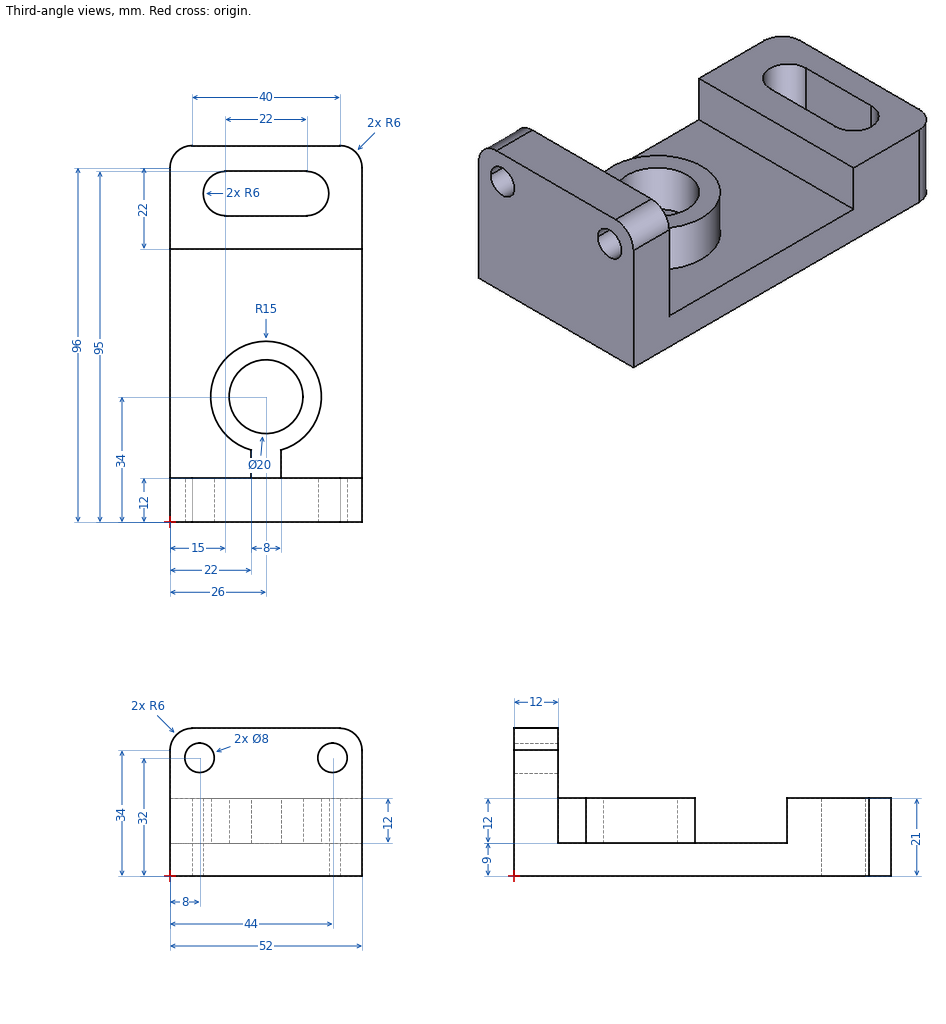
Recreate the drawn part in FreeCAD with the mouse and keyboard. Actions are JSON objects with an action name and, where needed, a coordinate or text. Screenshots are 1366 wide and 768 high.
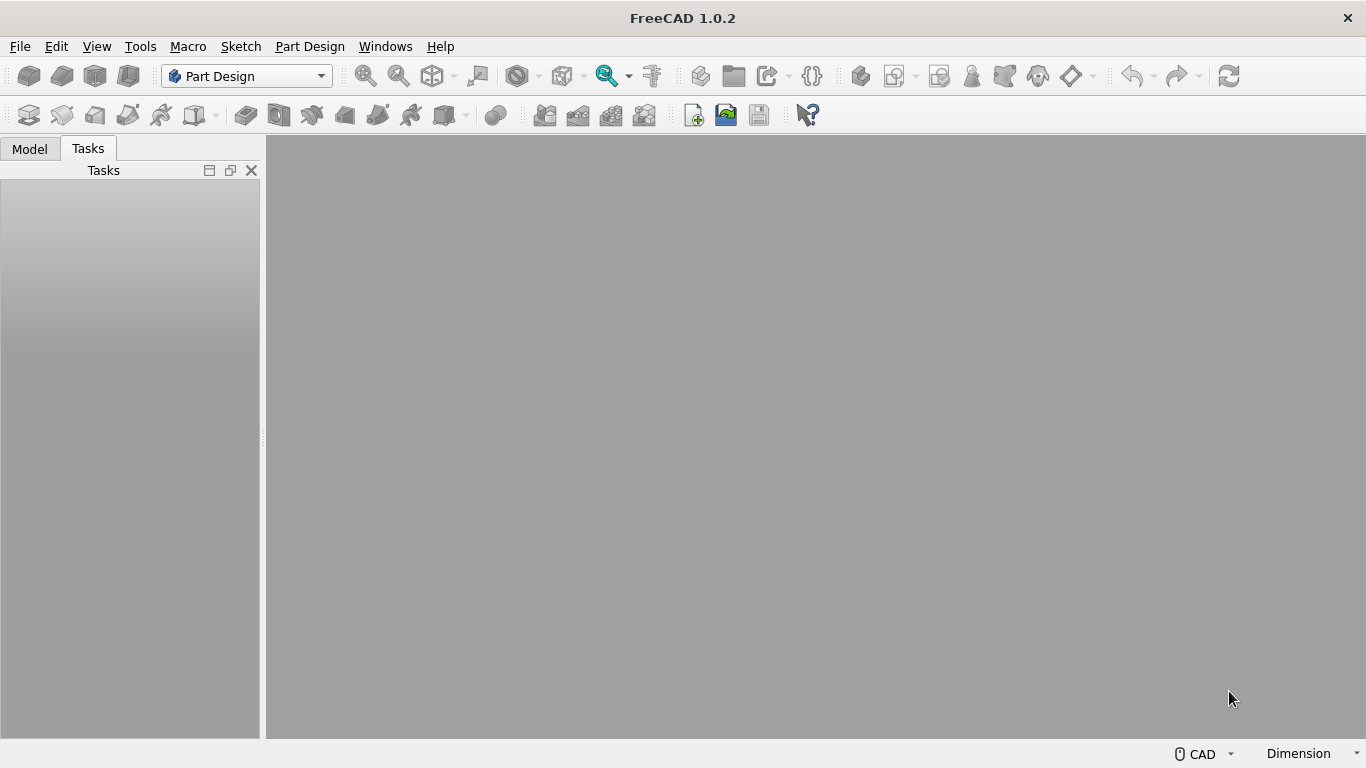
{"action": "left_click", "coordinate": [693, 116]}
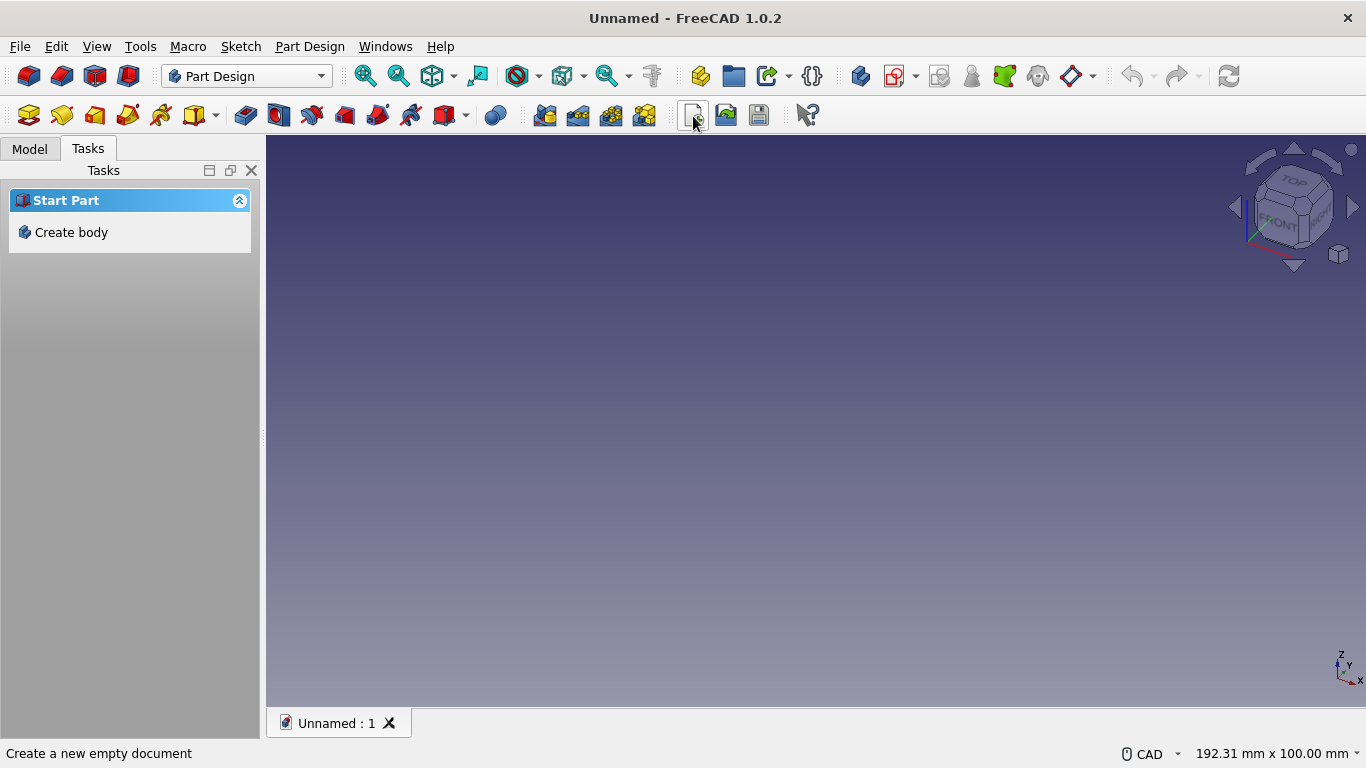
{"action": "left_click", "coordinate": [894, 76]}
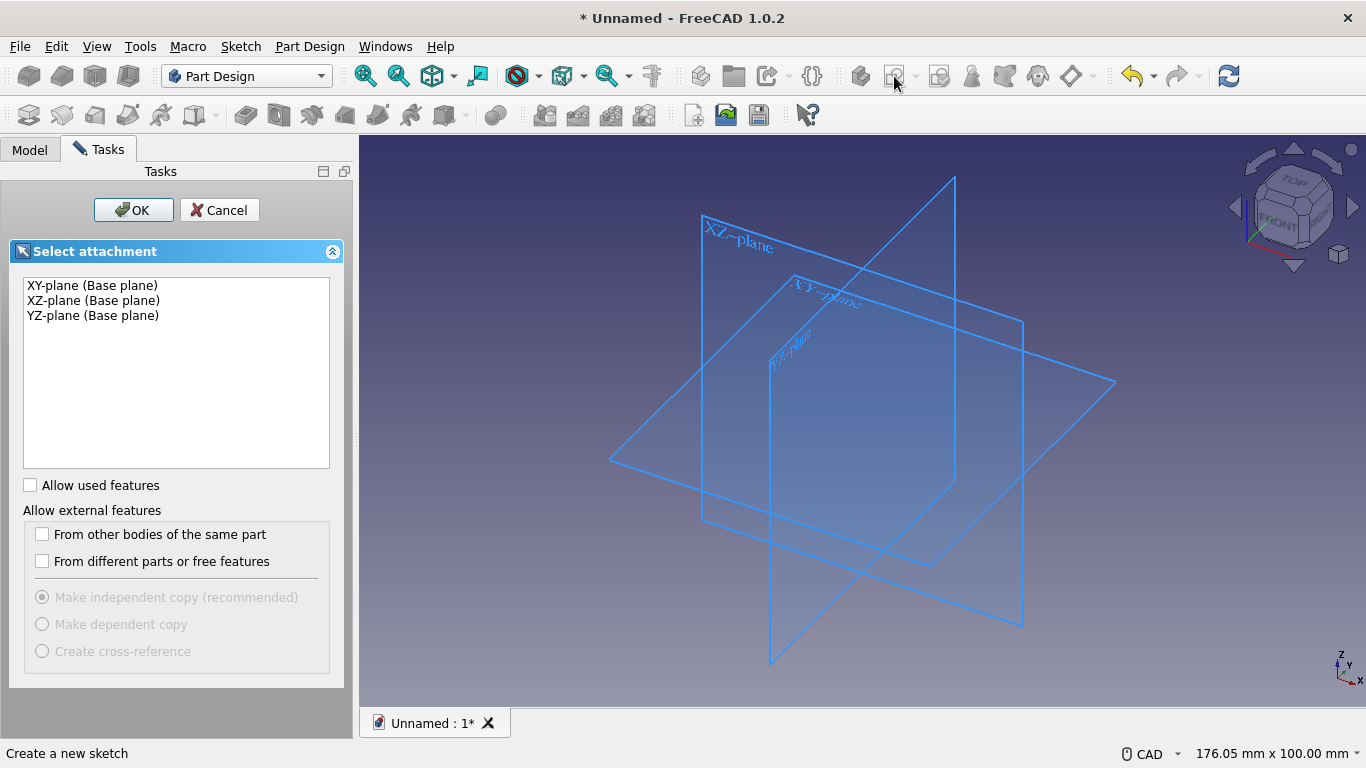
{"action": "left_click", "coordinate": [84, 286]}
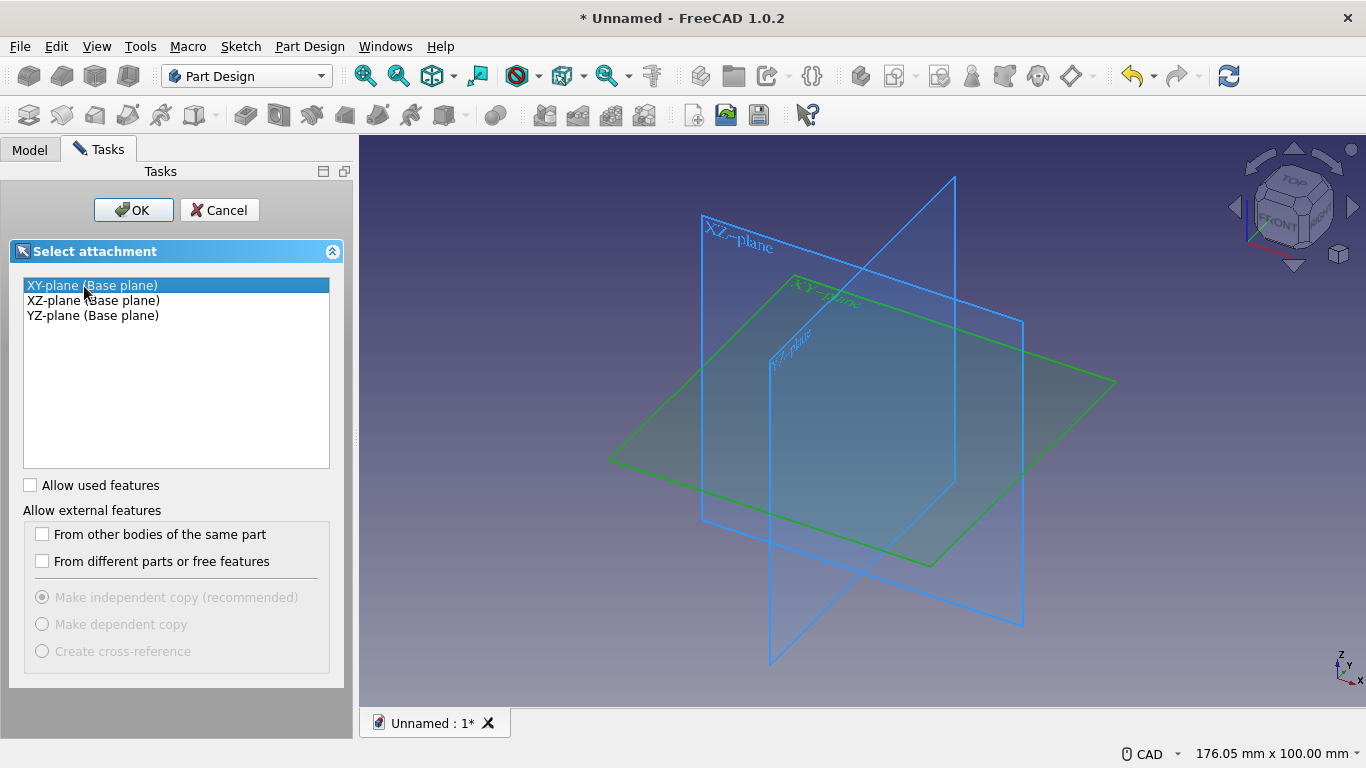
{"action": "left_click", "coordinate": [134, 210]}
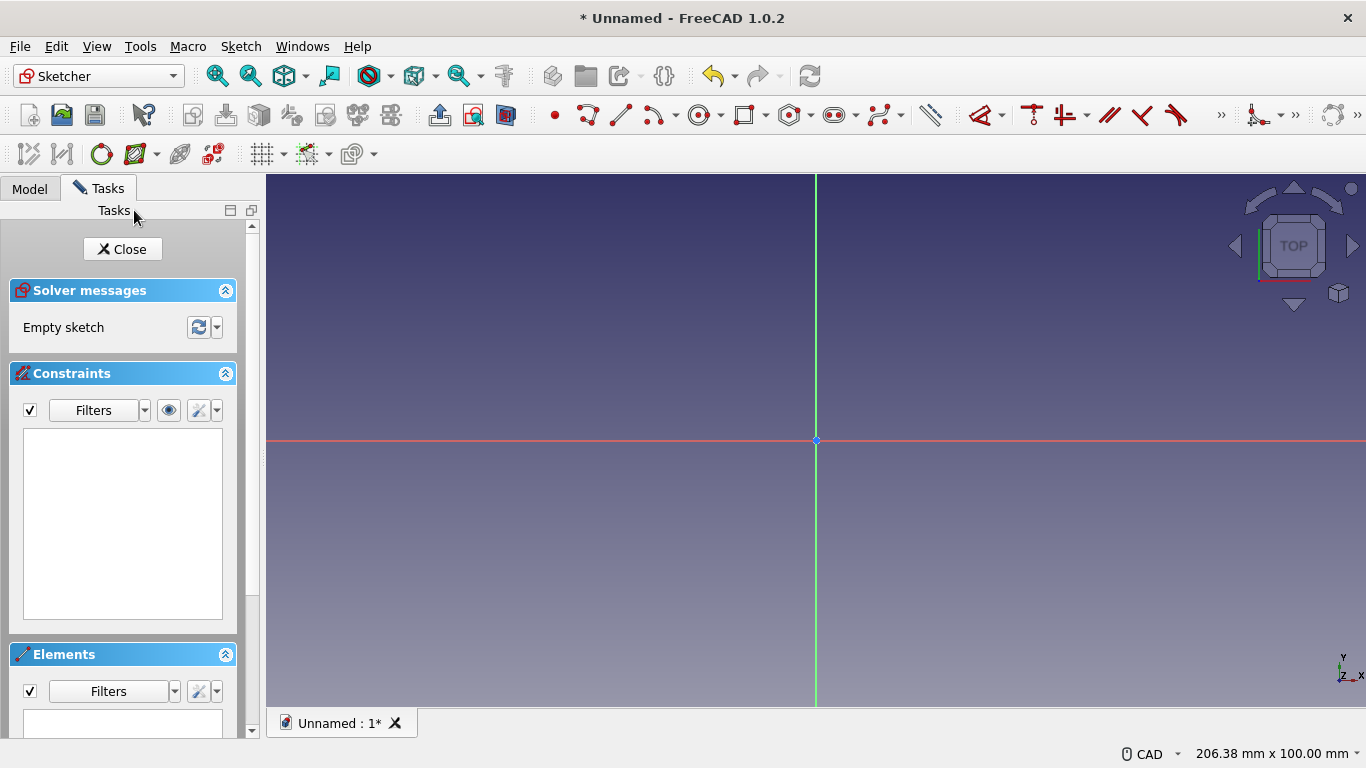
{"action": "scroll", "coordinate": [496, 679], "scroll_direction": "down", "scroll_amount": 3}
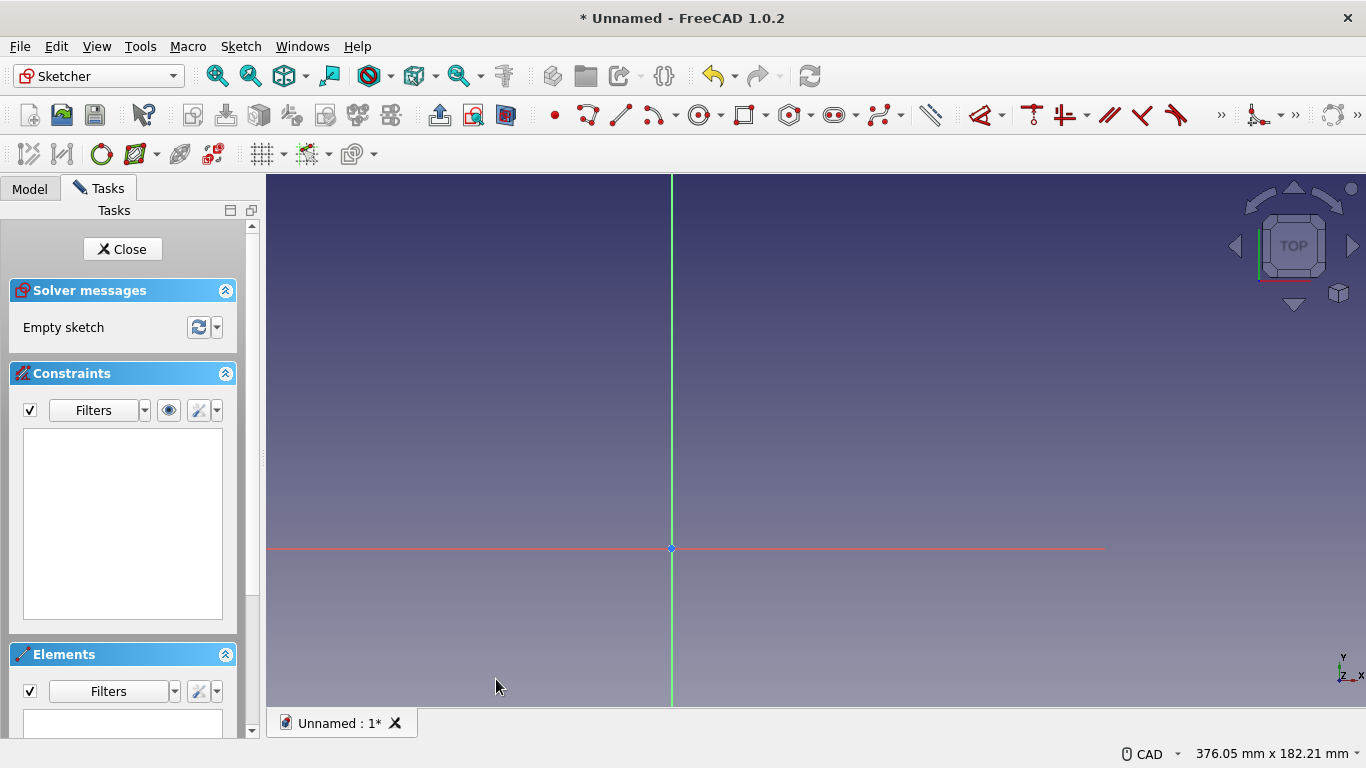
{"action": "left_click", "coordinate": [621, 116]}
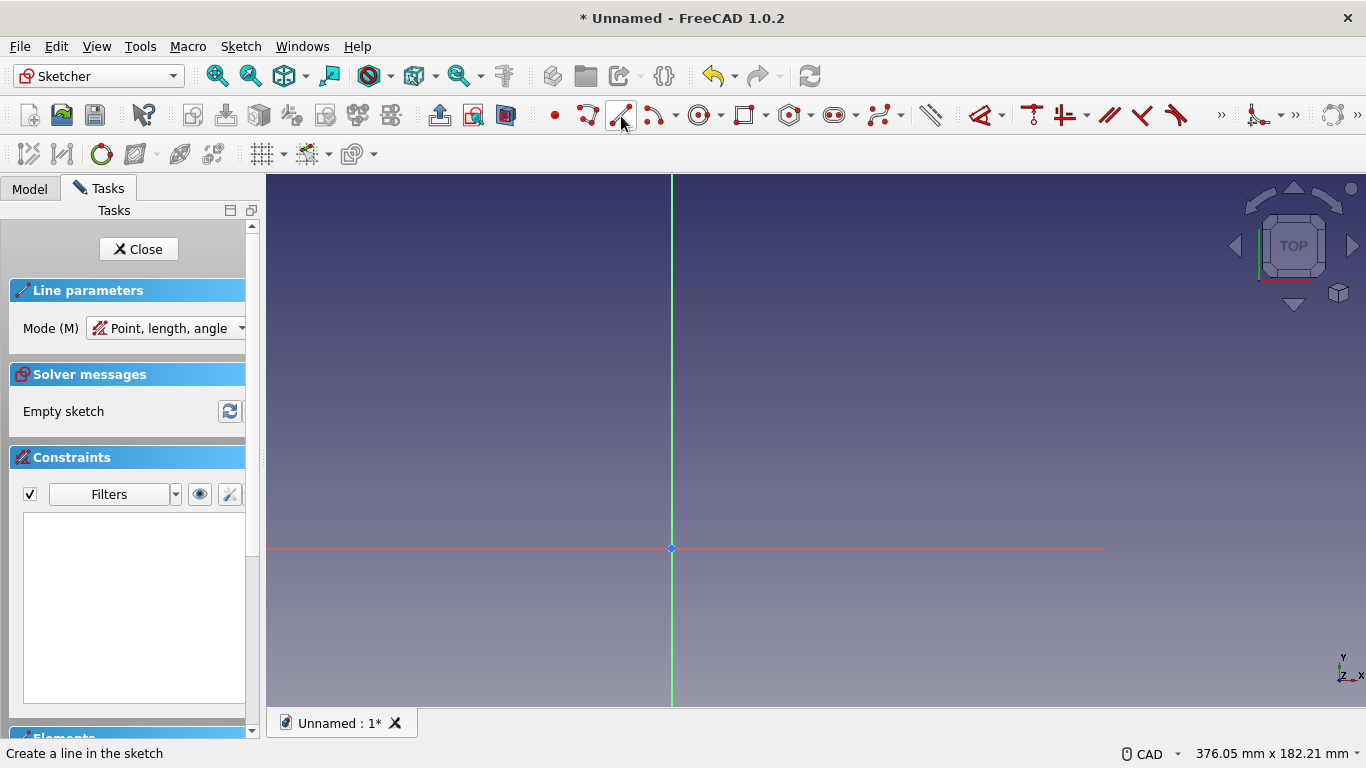
{"action": "left_click", "coordinate": [806, 250]}
{"action": "left_click", "coordinate": [689, 250]}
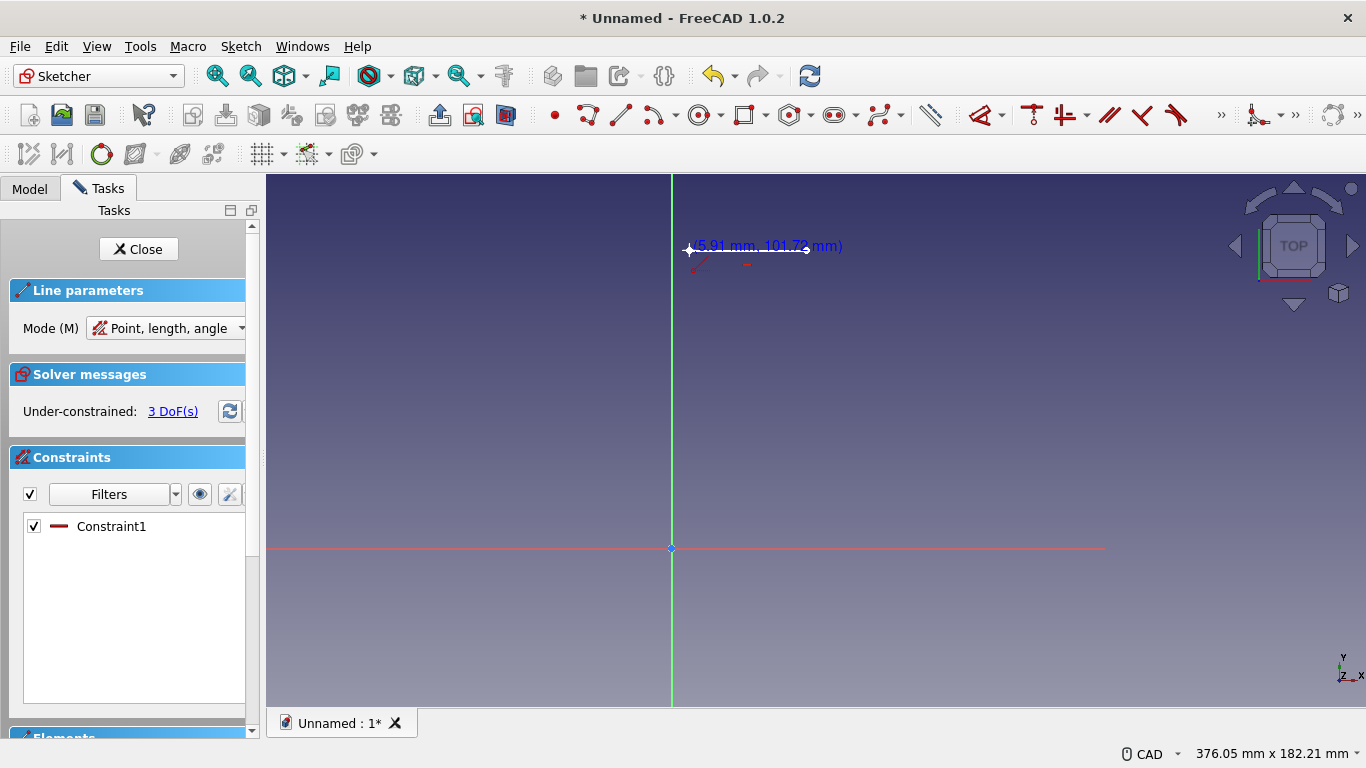
{"action": "key", "text": "g m"}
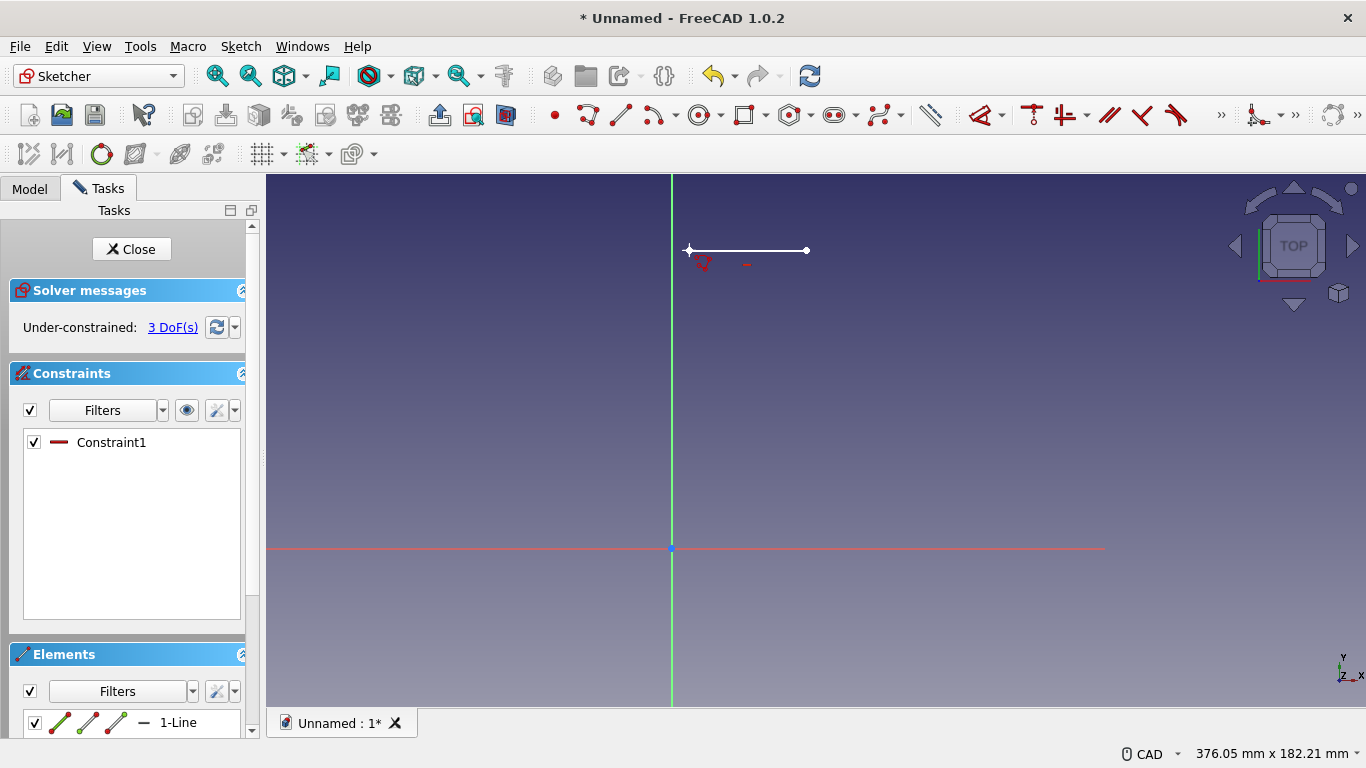
{"action": "left_click", "coordinate": [672, 268]}
{"action": "left_click", "coordinate": [672, 549]}
{"action": "left_click", "coordinate": [824, 540]}
{"action": "left_click", "coordinate": [824, 268]}
{"action": "right_click", "coordinate": [824, 268]}